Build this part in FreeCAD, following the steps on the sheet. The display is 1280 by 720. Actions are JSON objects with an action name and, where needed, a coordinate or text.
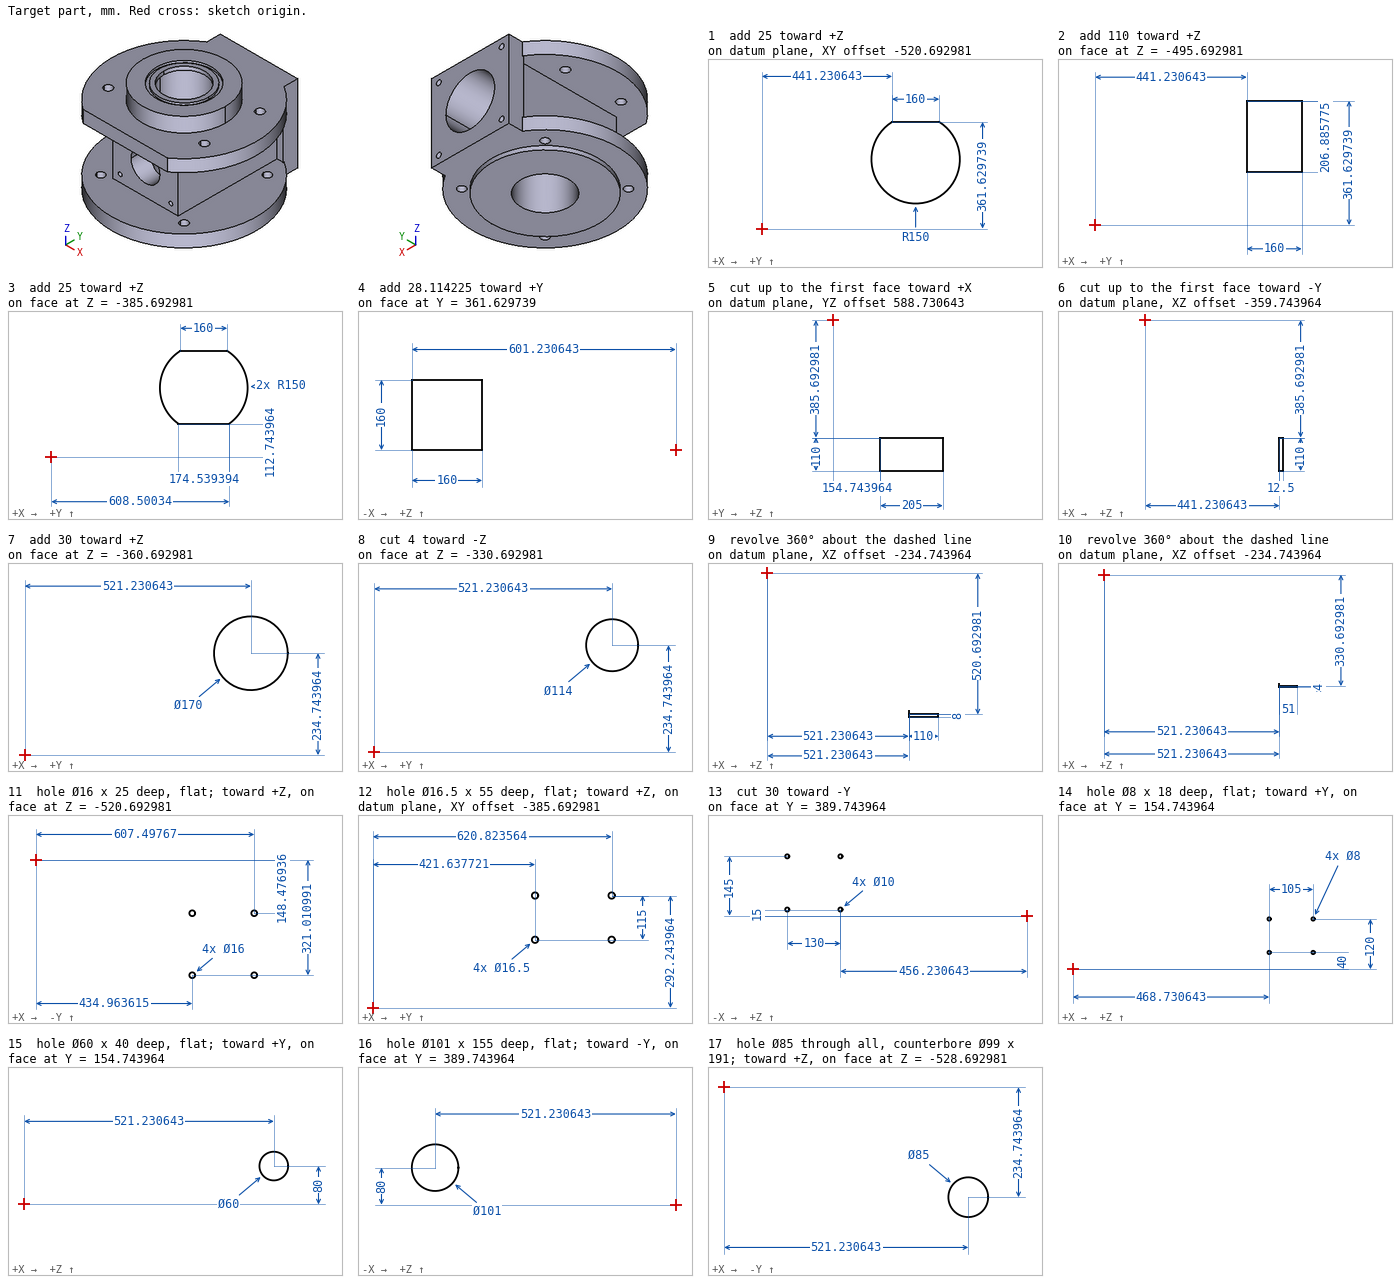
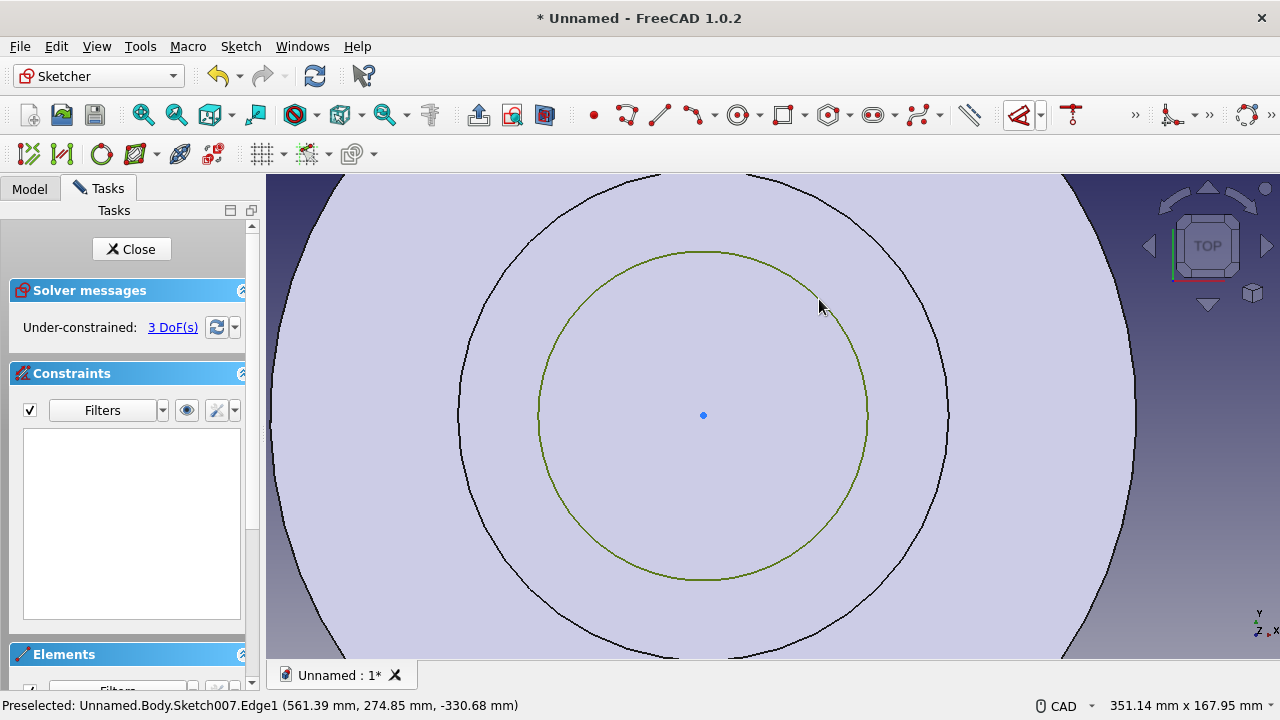
{"action": "left_click", "coordinate": [1040, 116]}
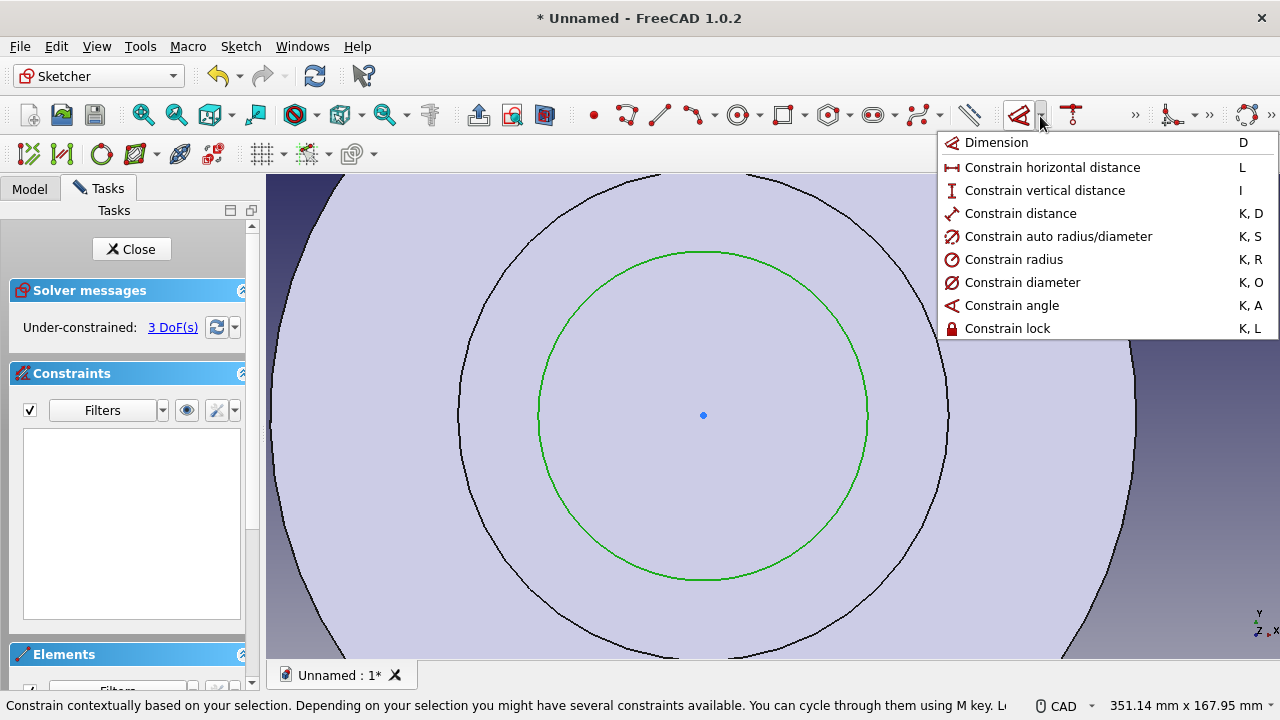
{"action": "left_click", "coordinate": [1108, 282]}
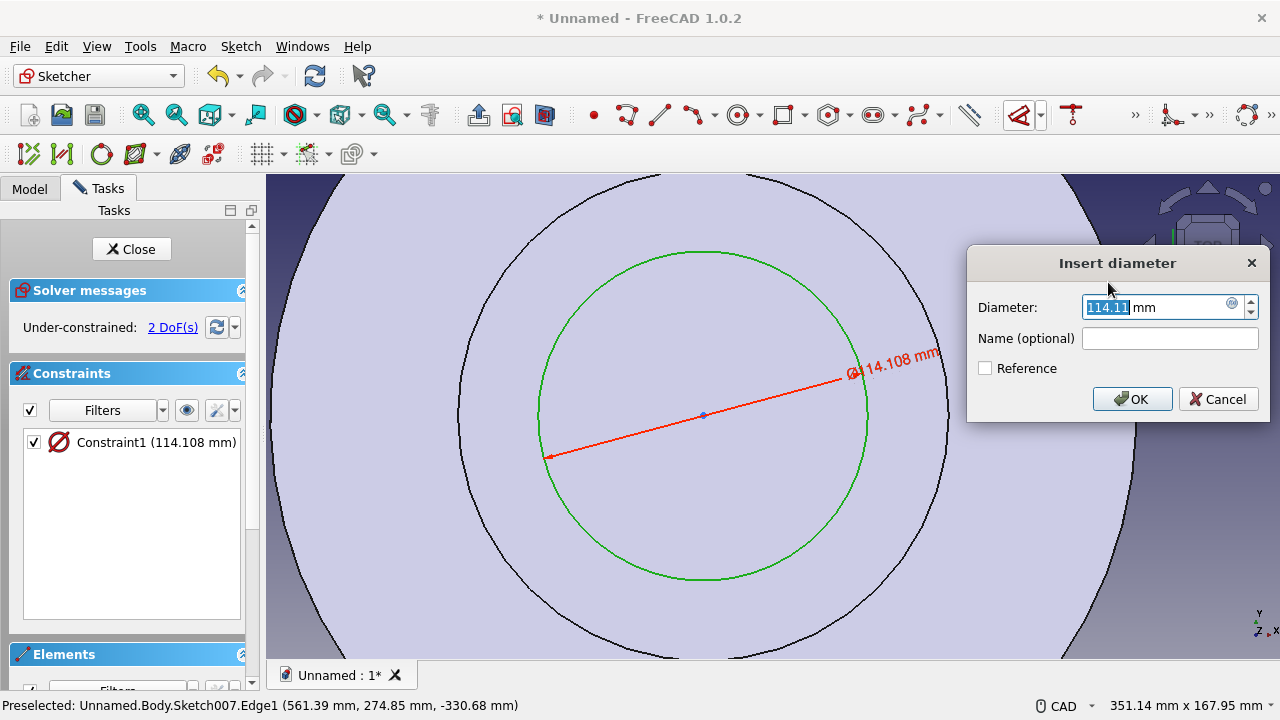
{"action": "type", "text": "114"}
{"action": "key", "text": "Return"}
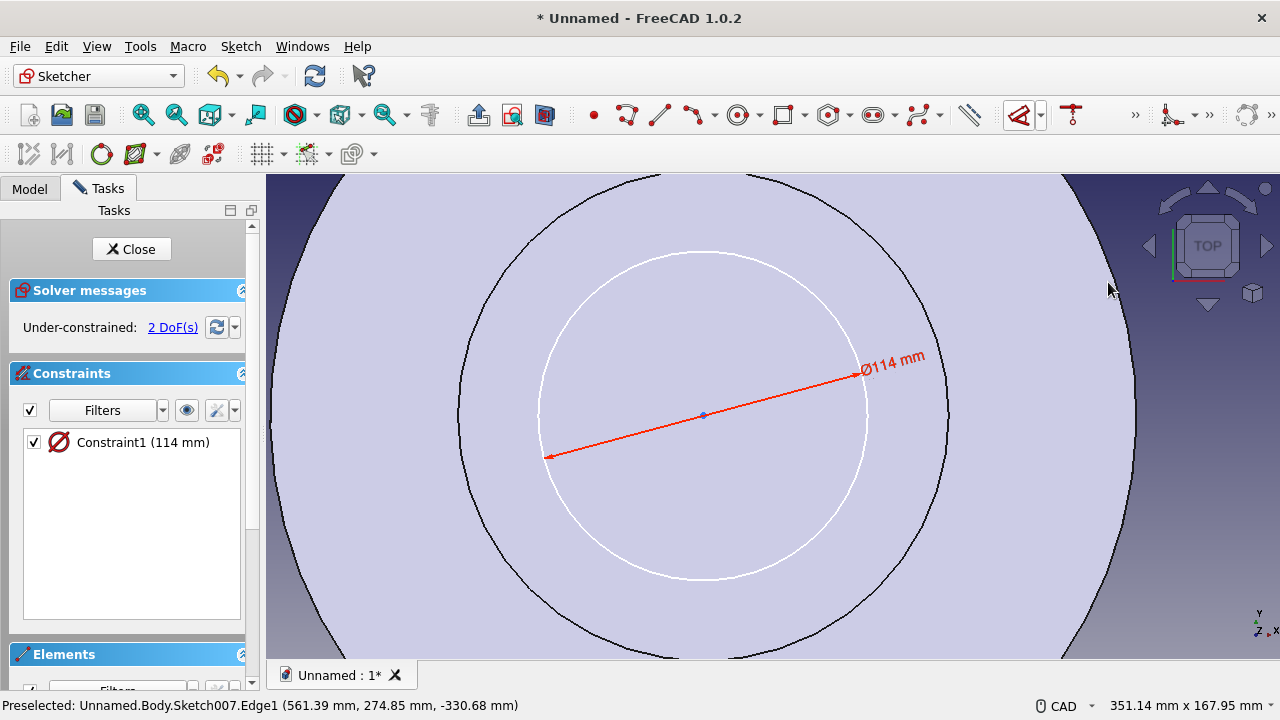
{"action": "left_click", "coordinate": [703, 416]}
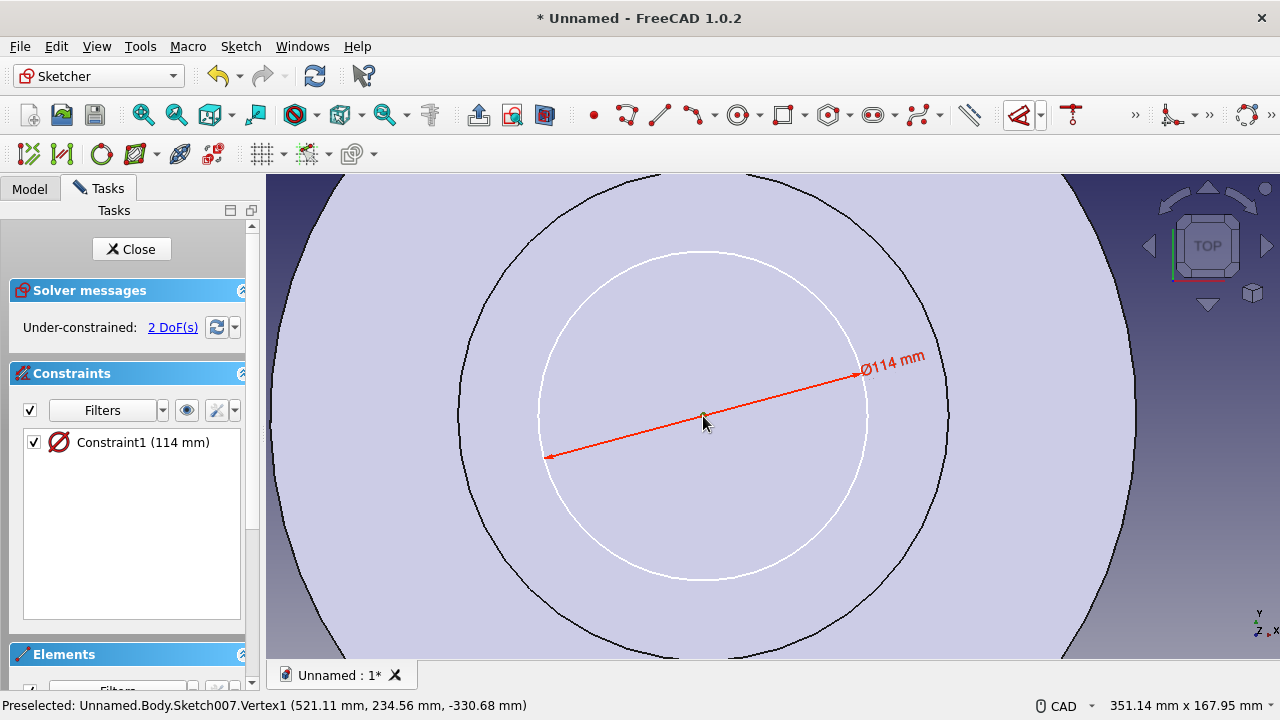
{"action": "left_click", "coordinate": [1040, 116]}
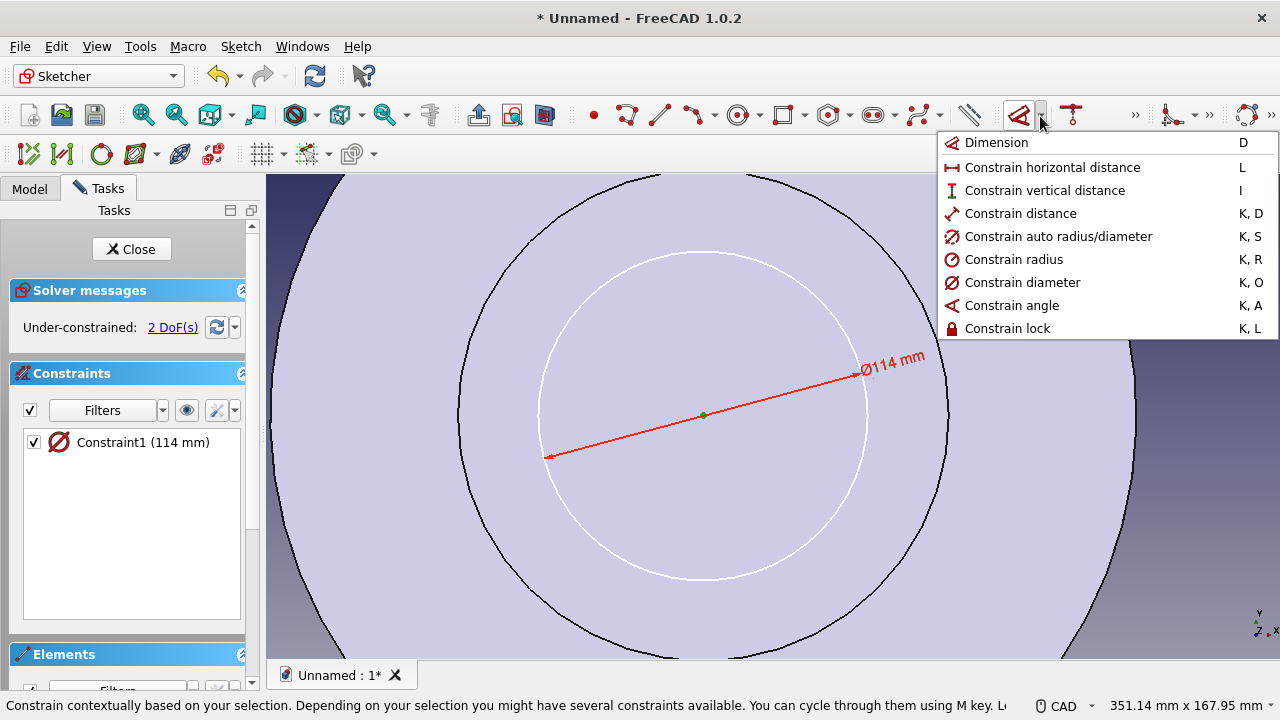
{"action": "left_click", "coordinate": [1108, 168]}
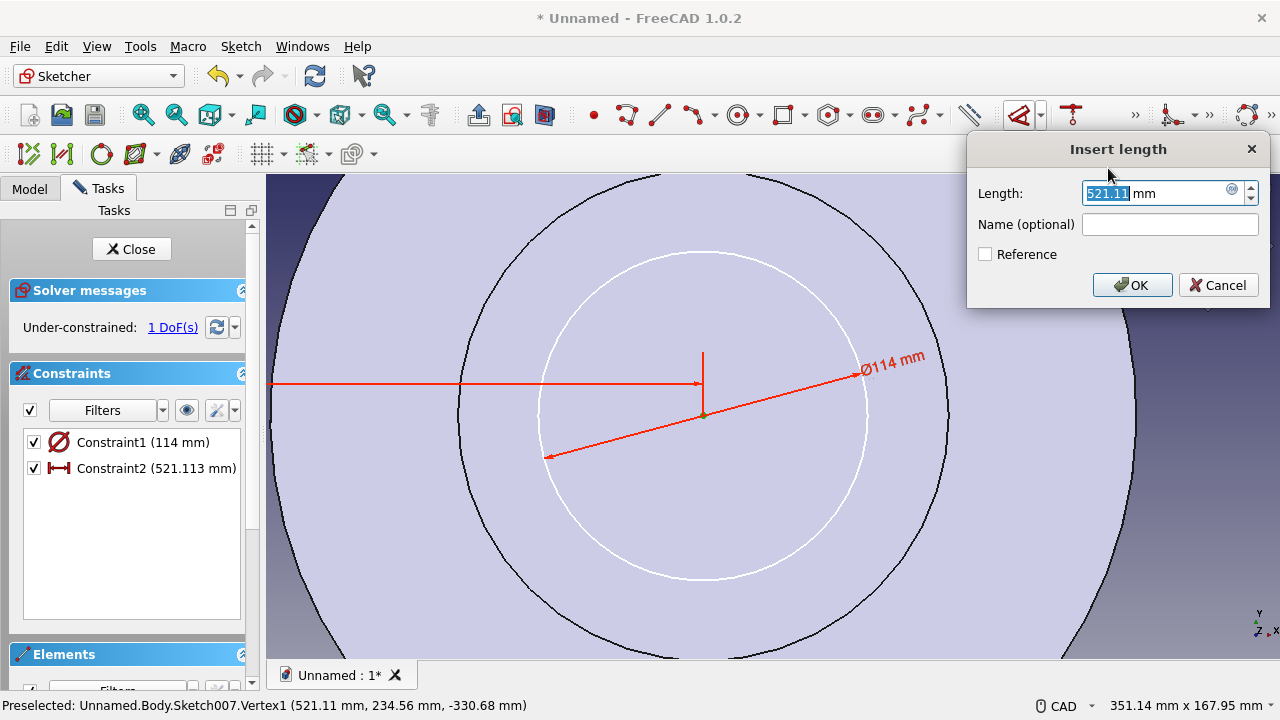
{"action": "type", "text": "521.230643"}
{"action": "key", "text": "Return"}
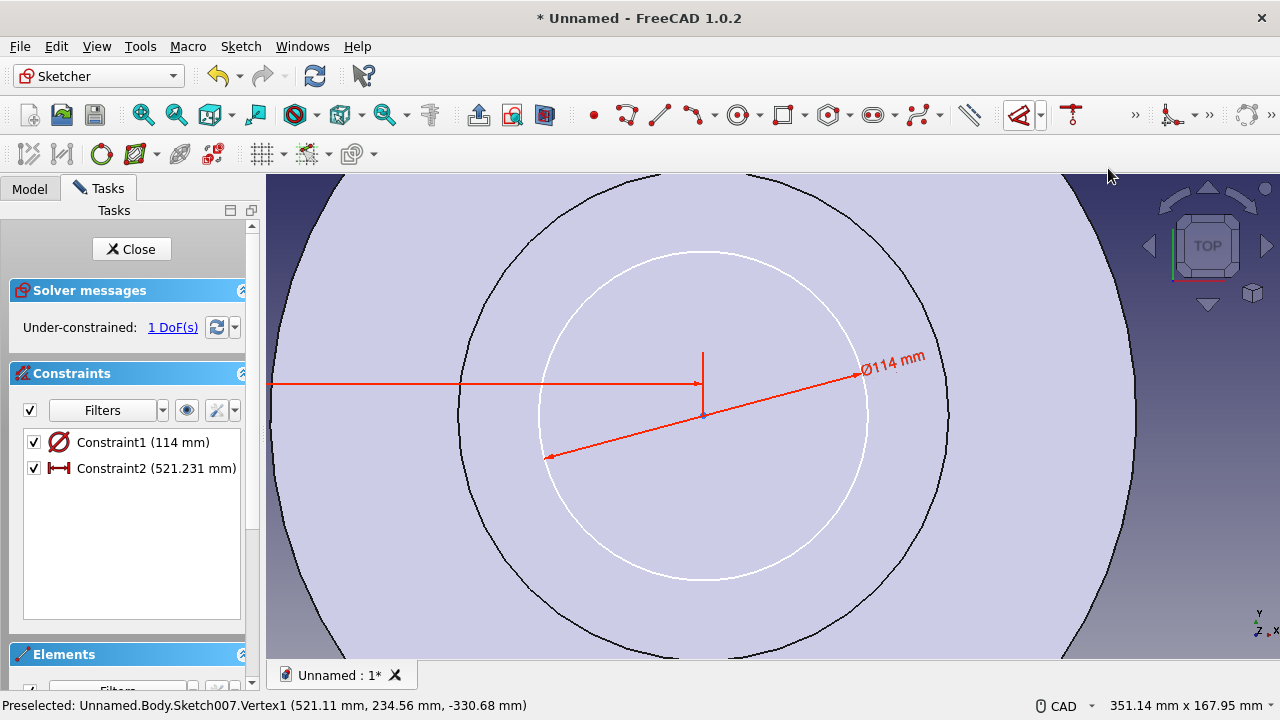
{"action": "left_click", "coordinate": [703, 416]}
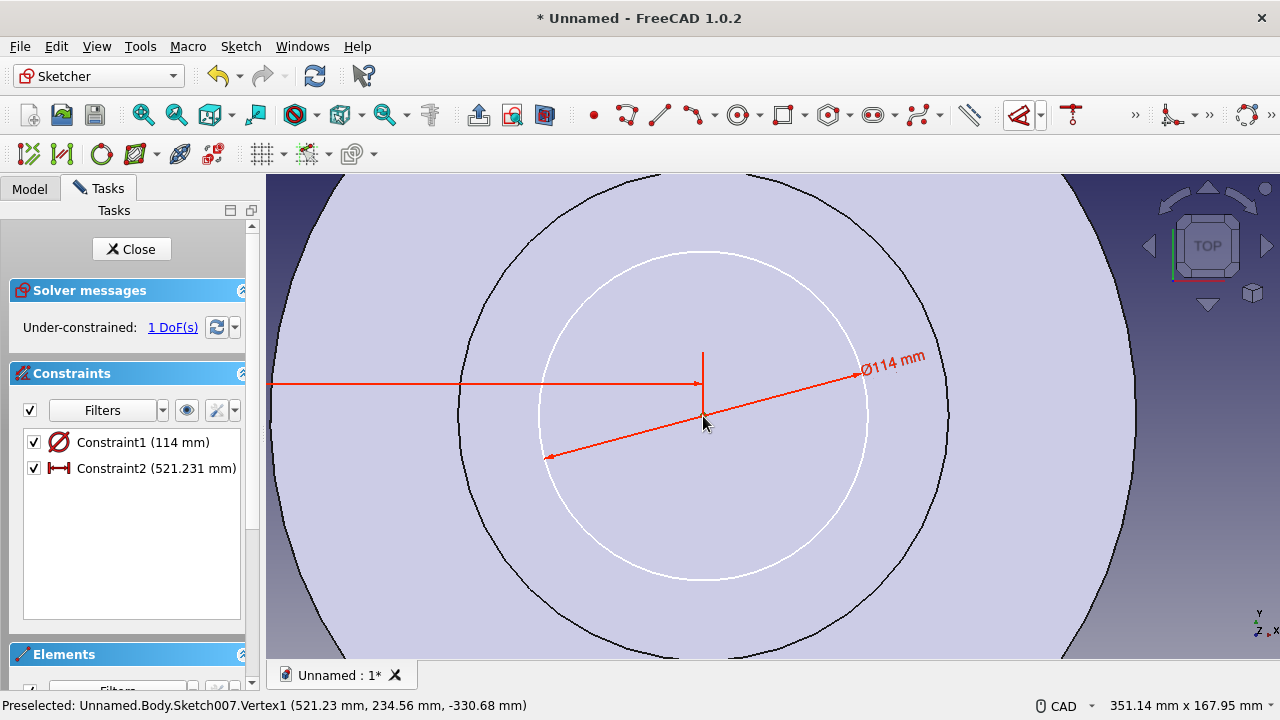
{"action": "left_click", "coordinate": [1040, 116]}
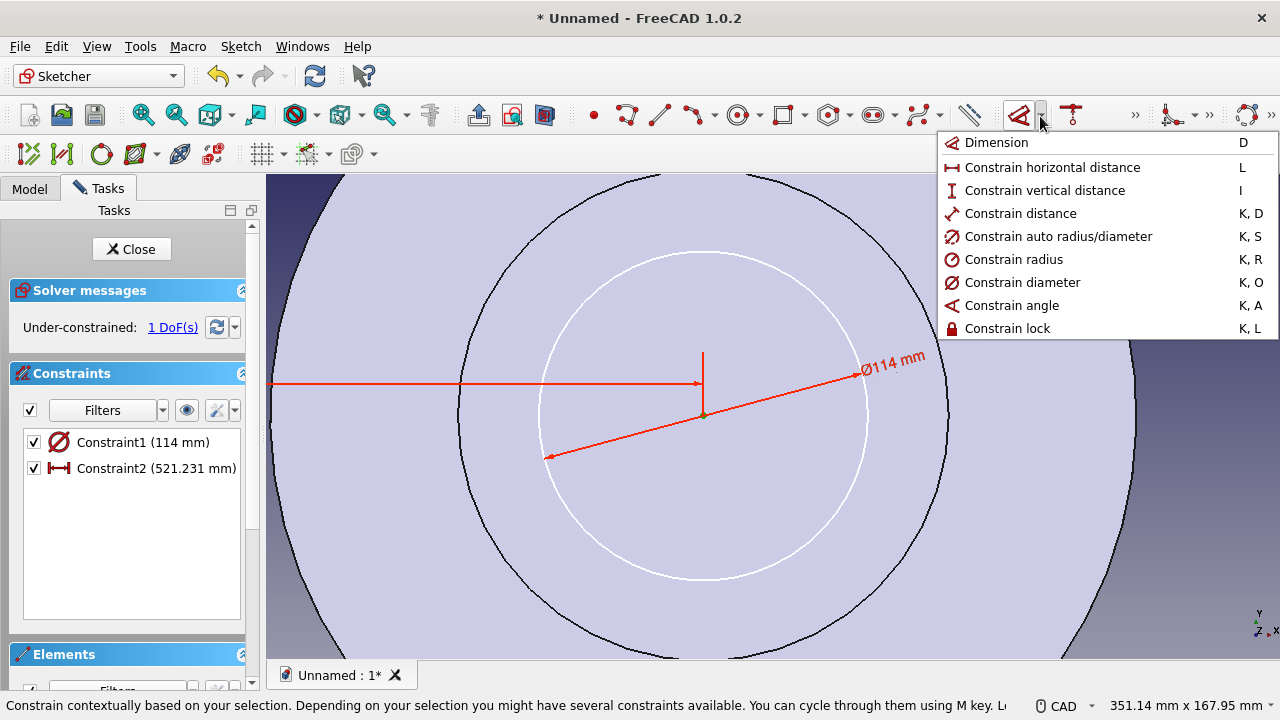
{"action": "left_click", "coordinate": [1108, 190]}